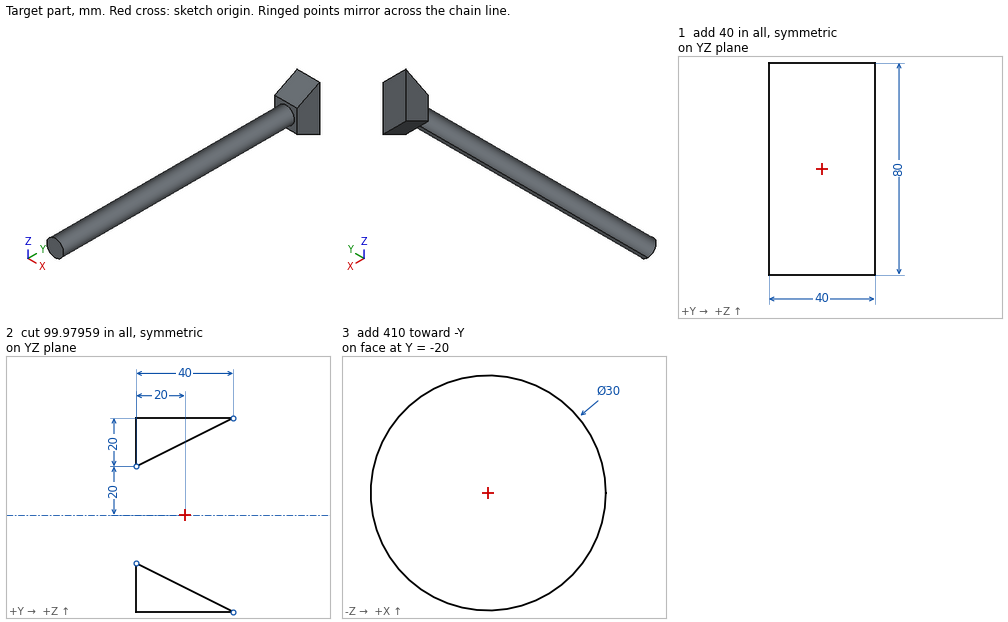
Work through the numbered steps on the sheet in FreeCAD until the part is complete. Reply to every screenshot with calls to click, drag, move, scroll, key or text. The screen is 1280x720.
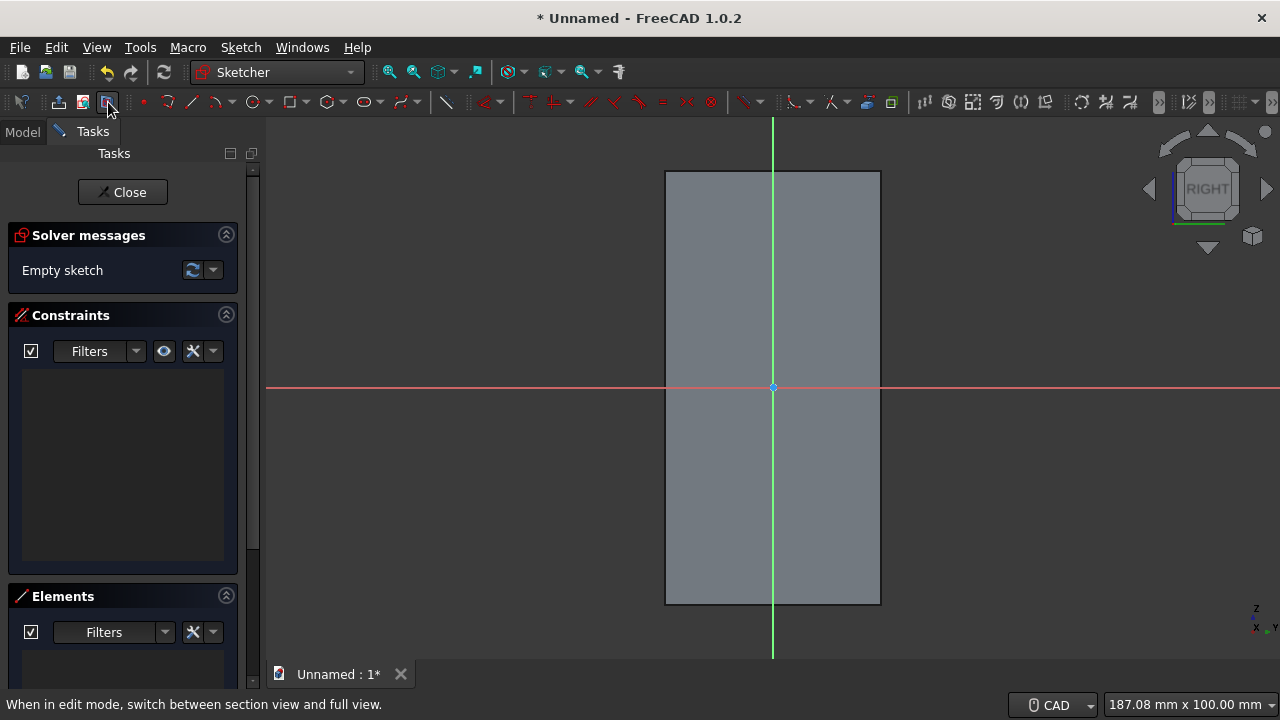
click(665, 280)
click(881, 171)
click(665, 171)
click(665, 281)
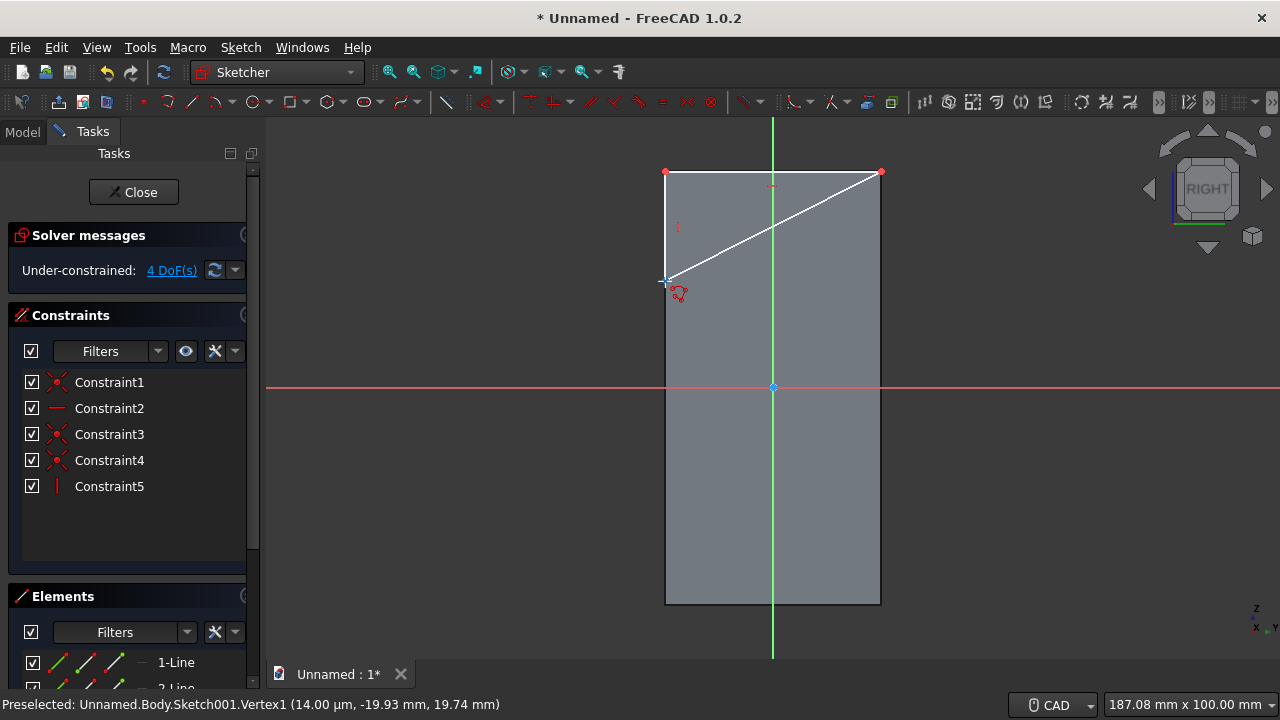
click(665, 496)
click(665, 605)
click(881, 605)
click(665, 497)
key(Escape)
key(Escape)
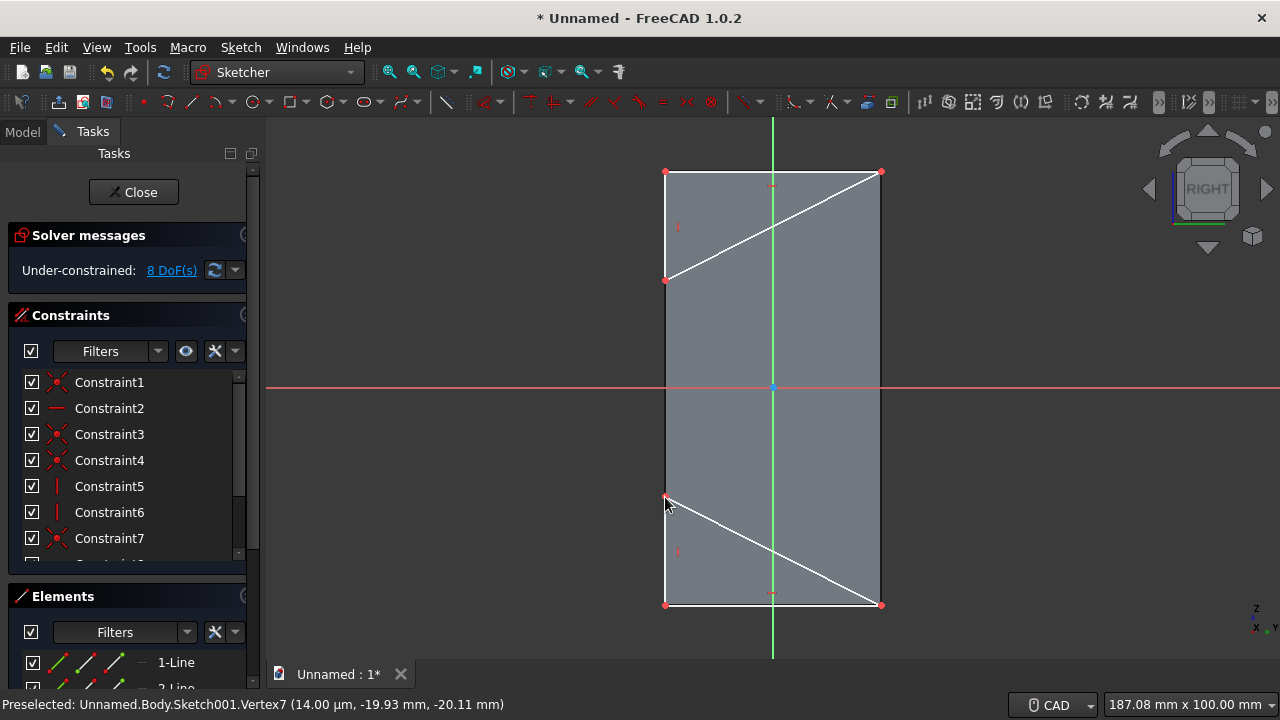
click(665, 281)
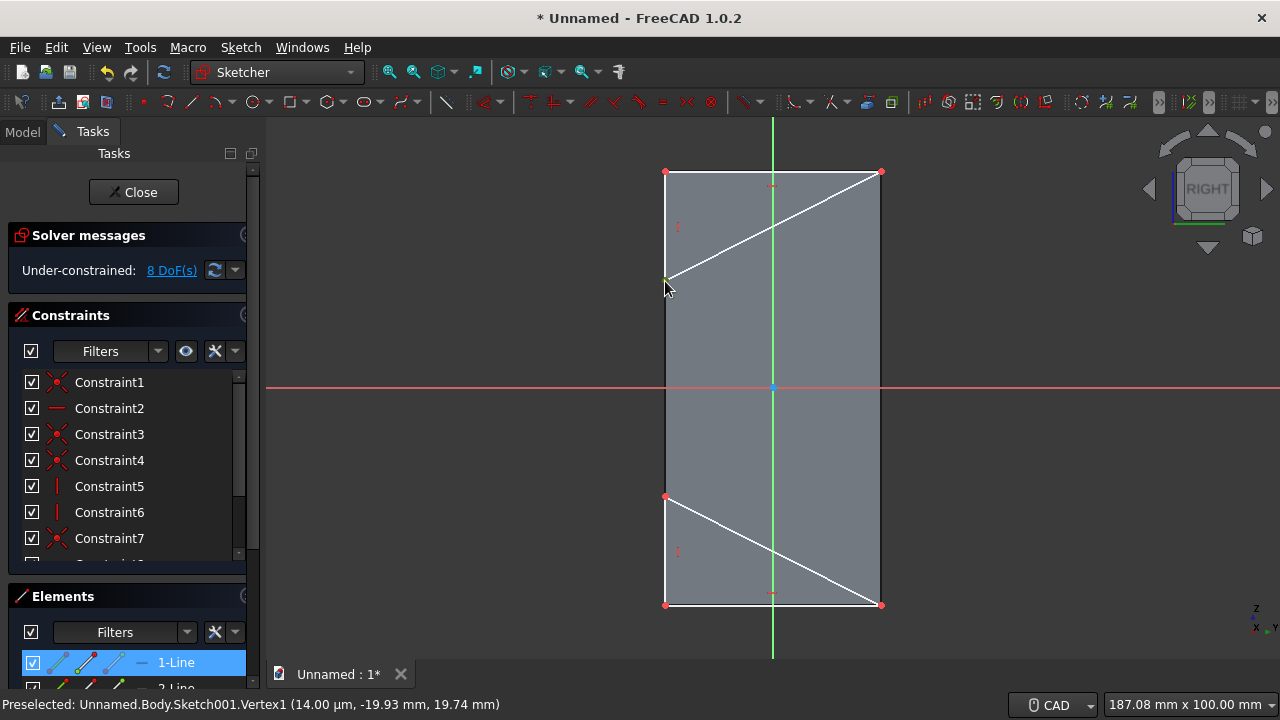
click(665, 497)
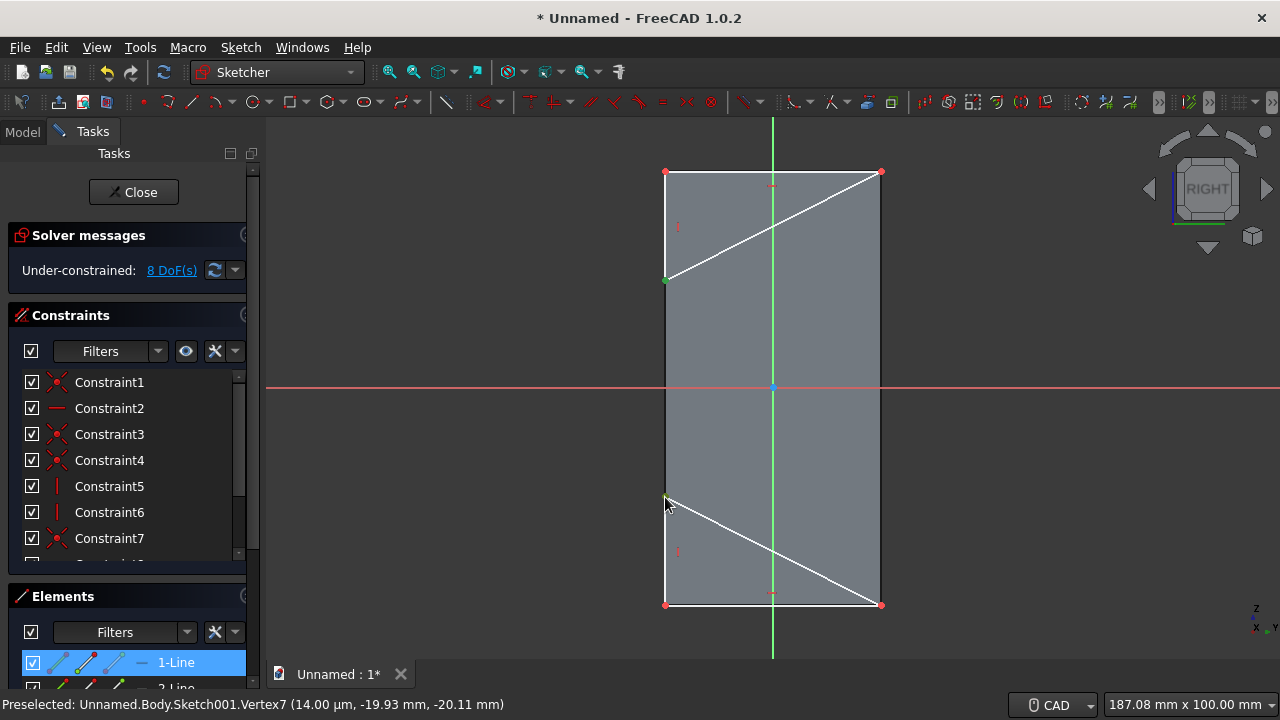
click(353, 388)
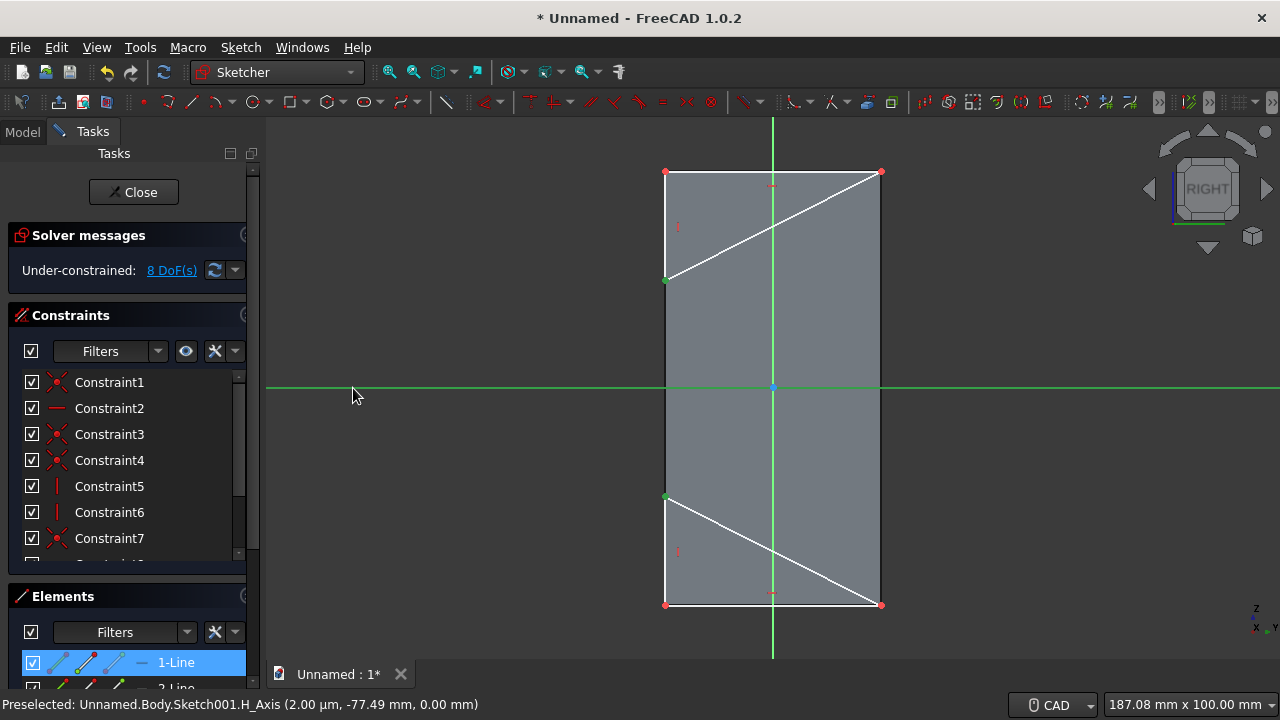
key(s)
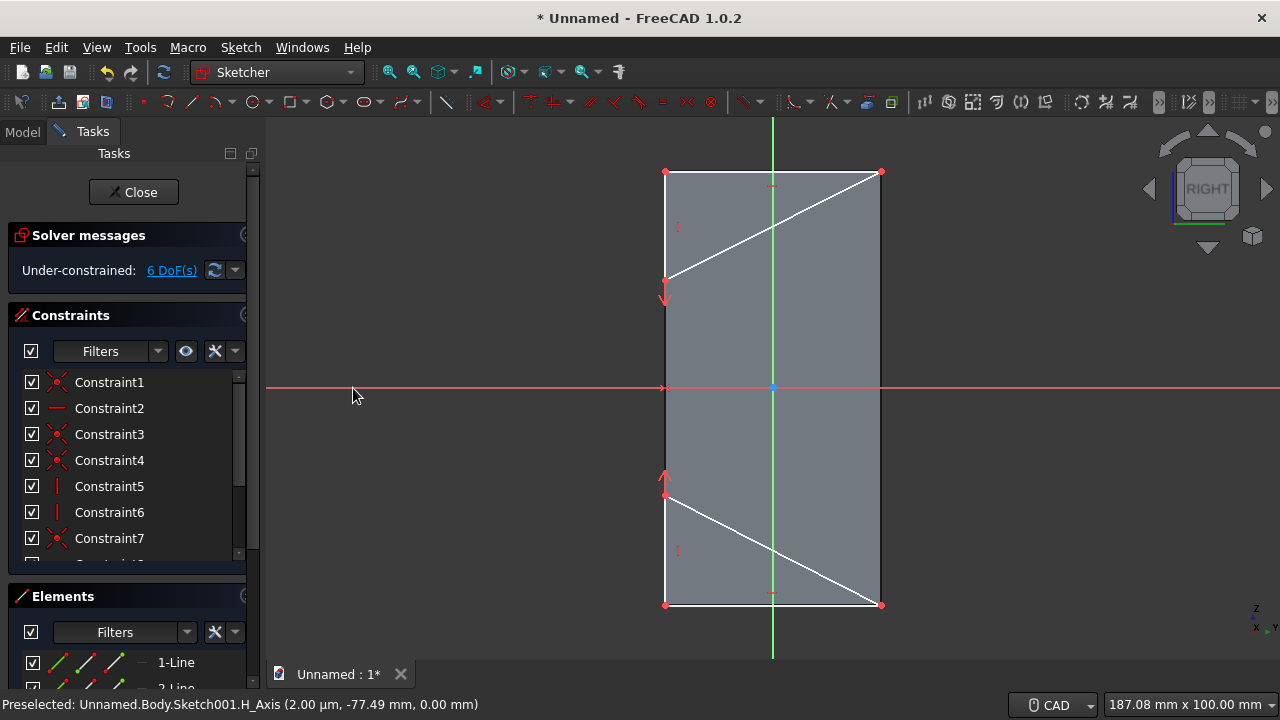
click(881, 172)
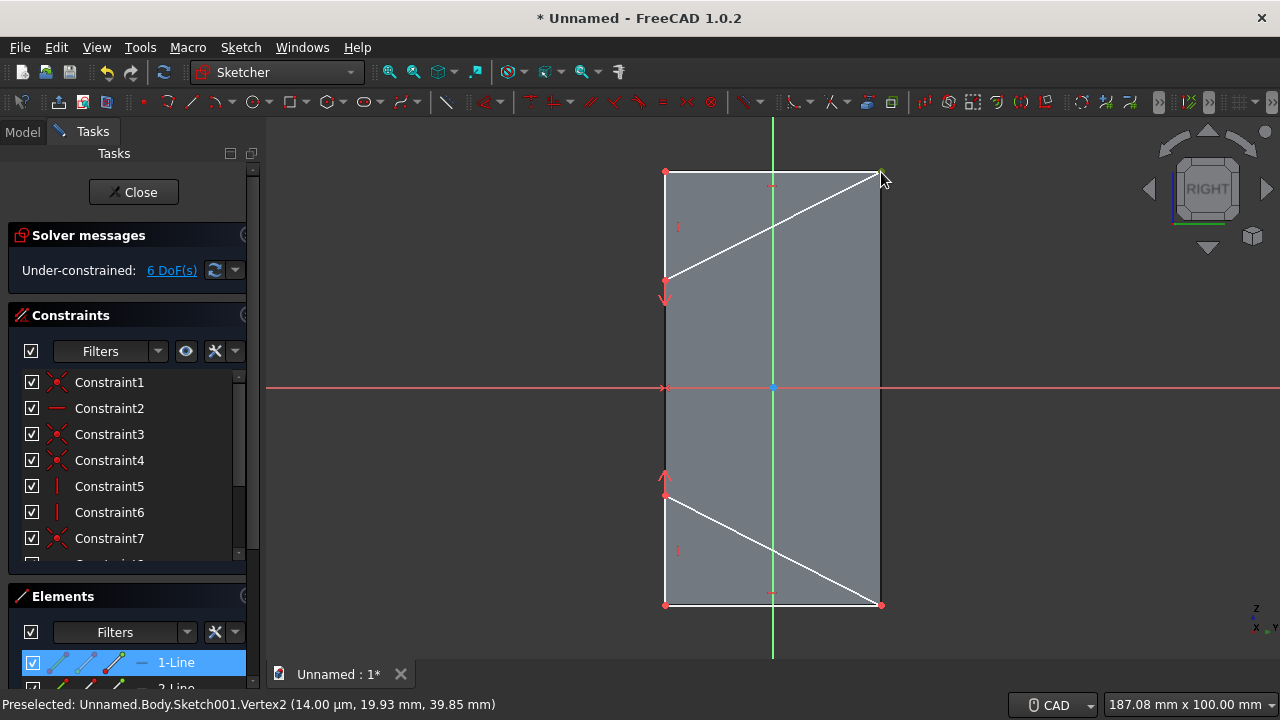
click(881, 606)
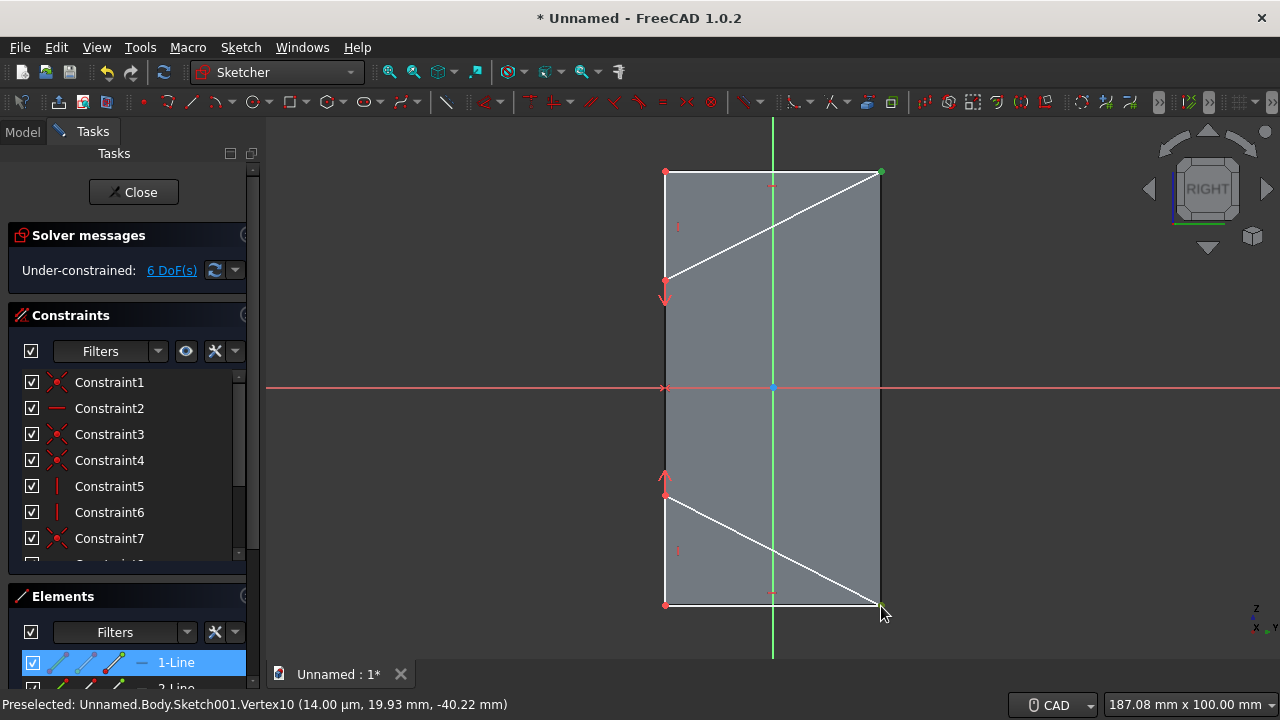
click(353, 388)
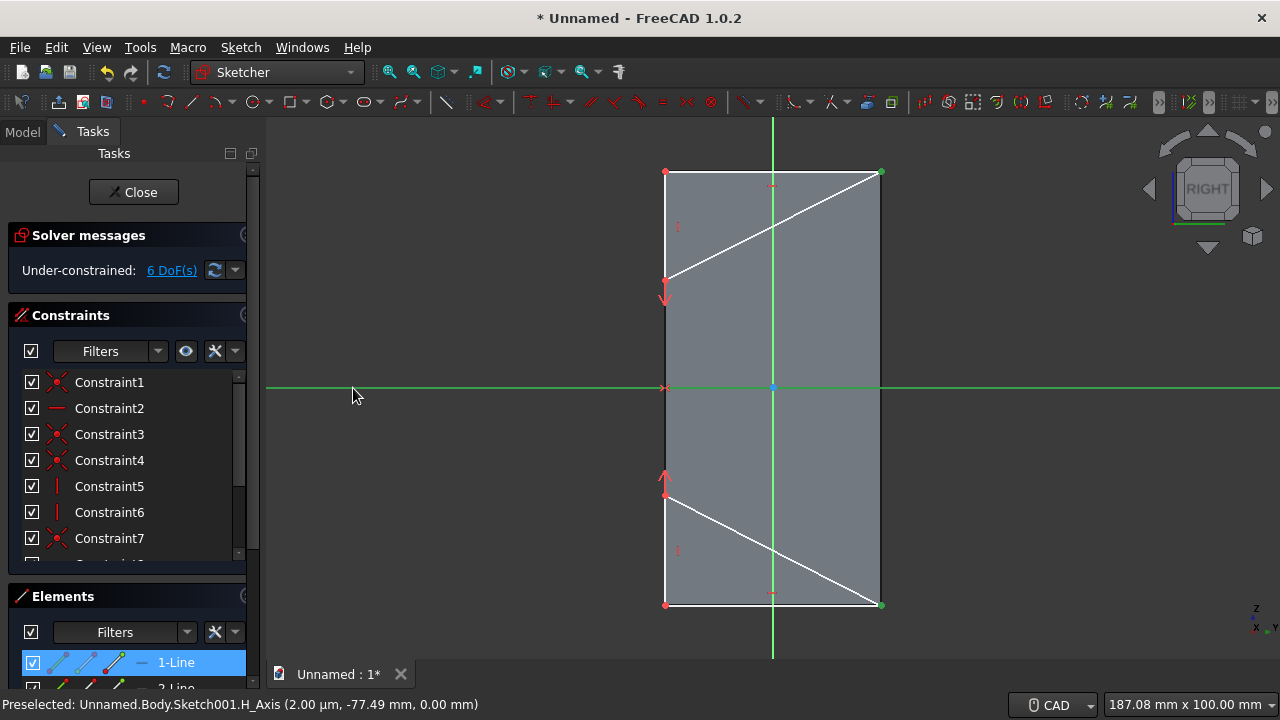
click(688, 102)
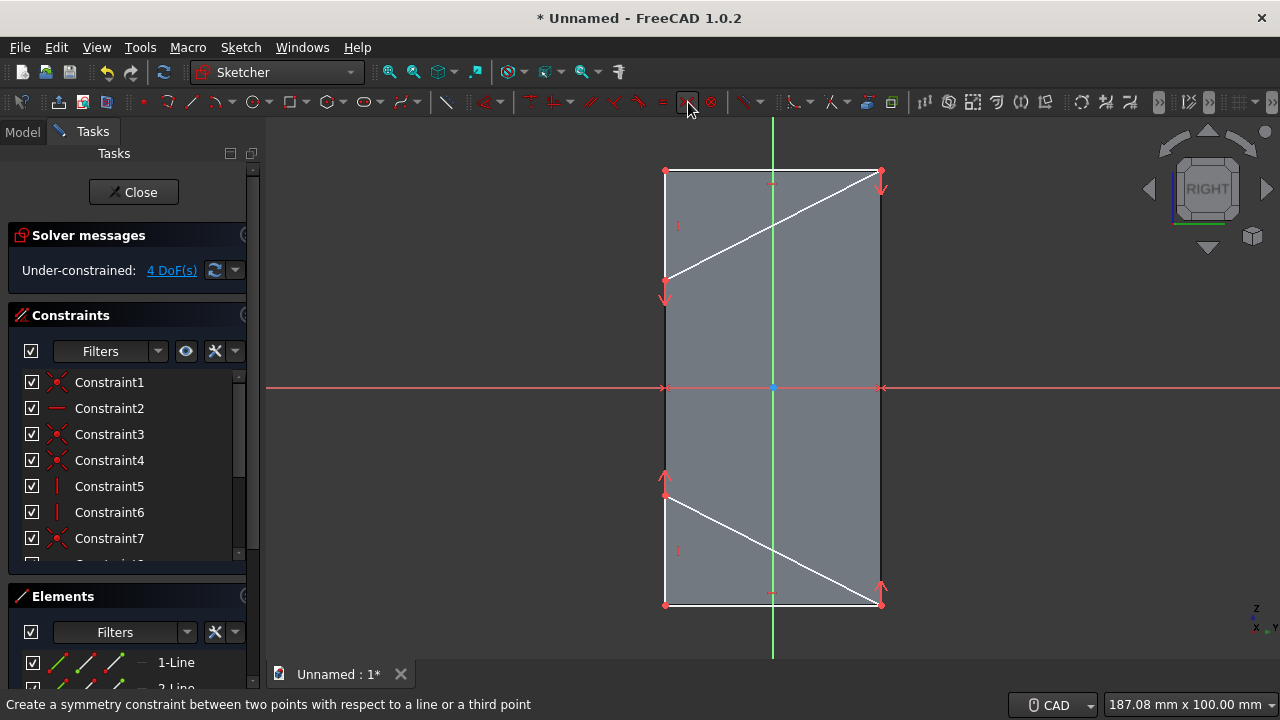
click(816, 170)